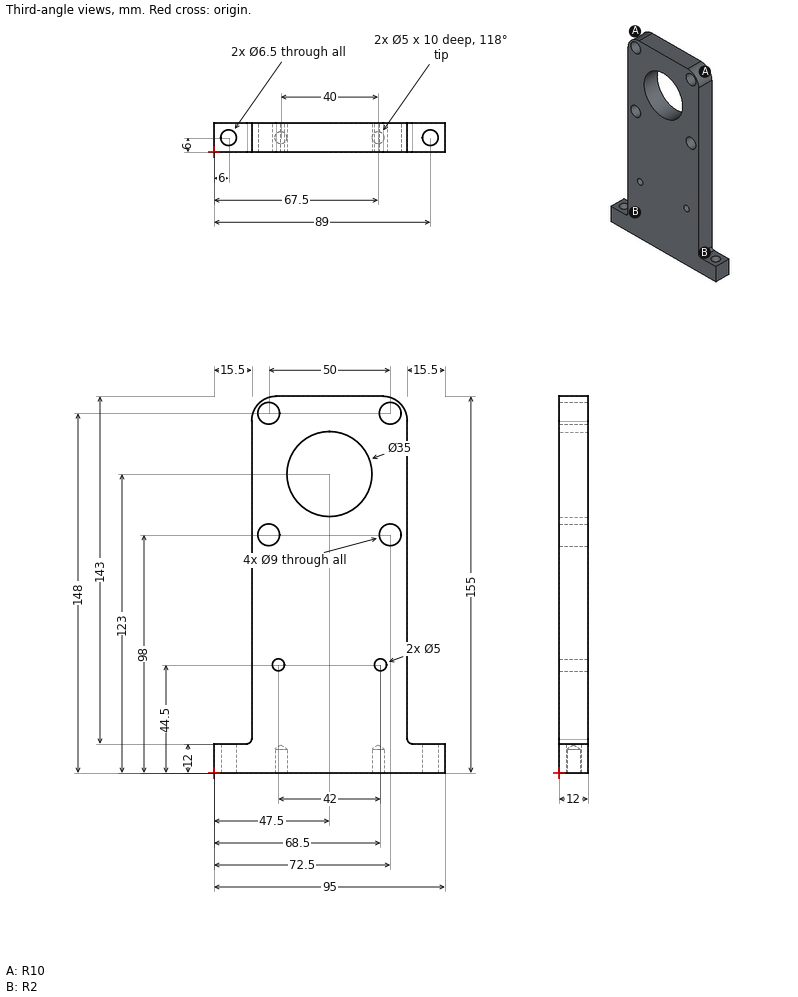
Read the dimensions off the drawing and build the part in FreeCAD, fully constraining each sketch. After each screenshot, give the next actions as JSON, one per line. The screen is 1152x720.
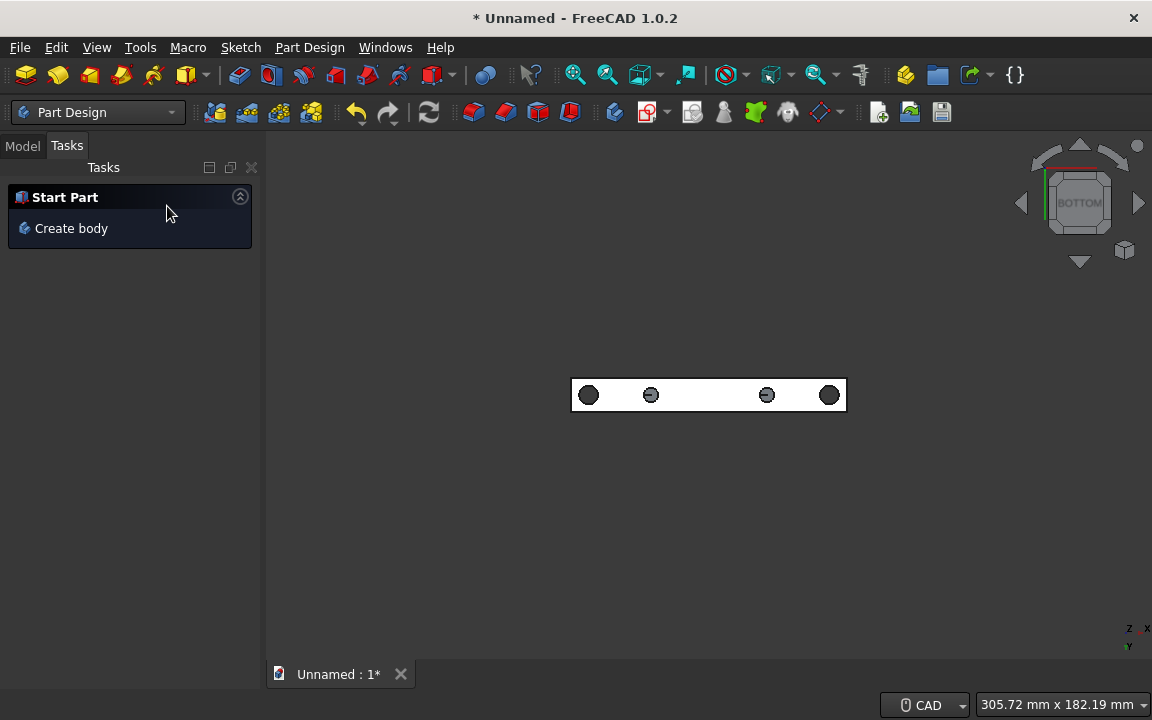
{"action": "key", "text": "0"}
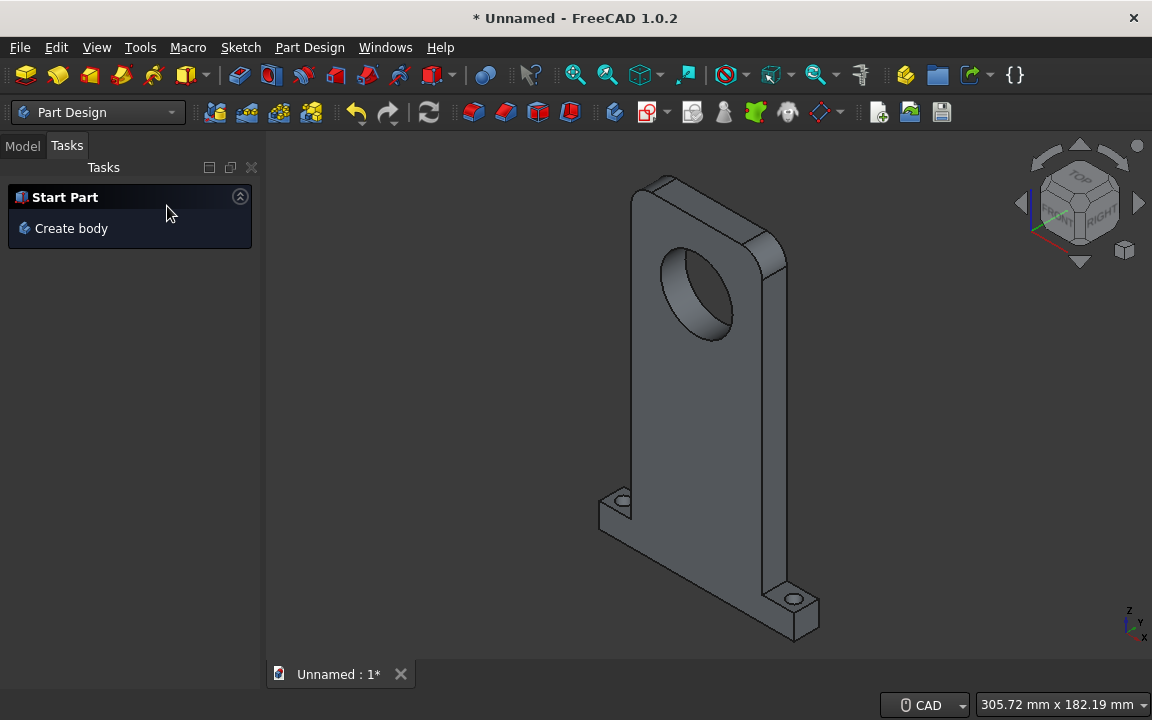
{"action": "key", "text": "2"}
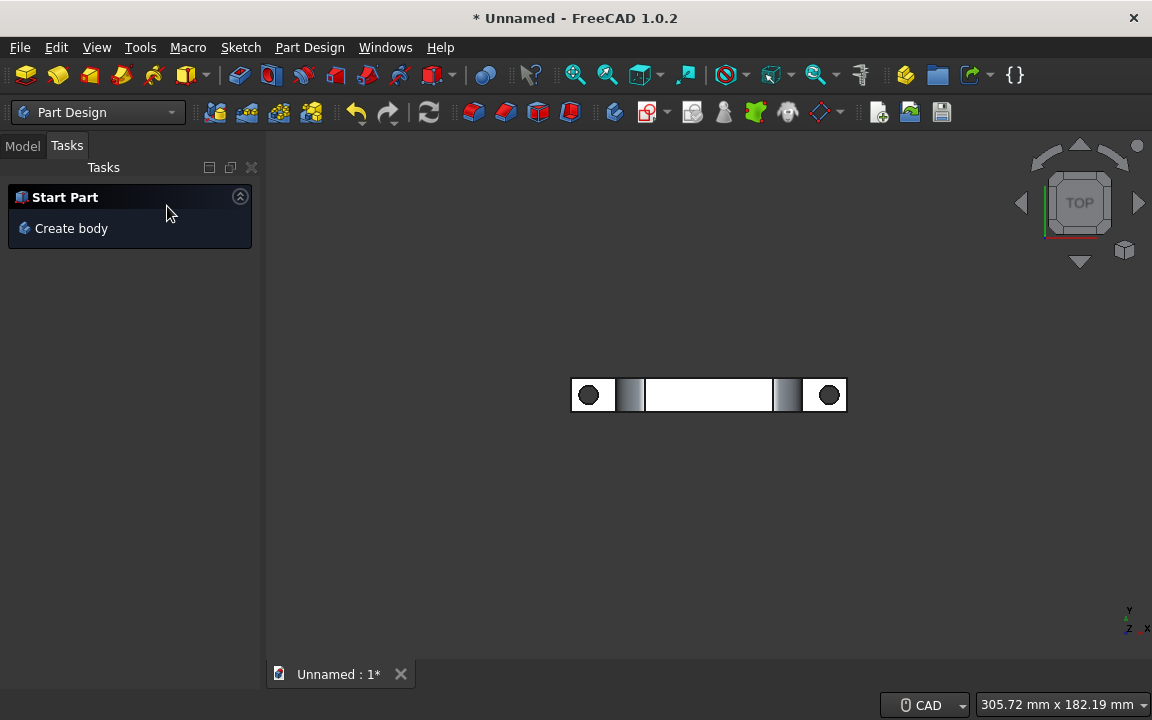
{"action": "left_click", "coordinate": [576, 76]}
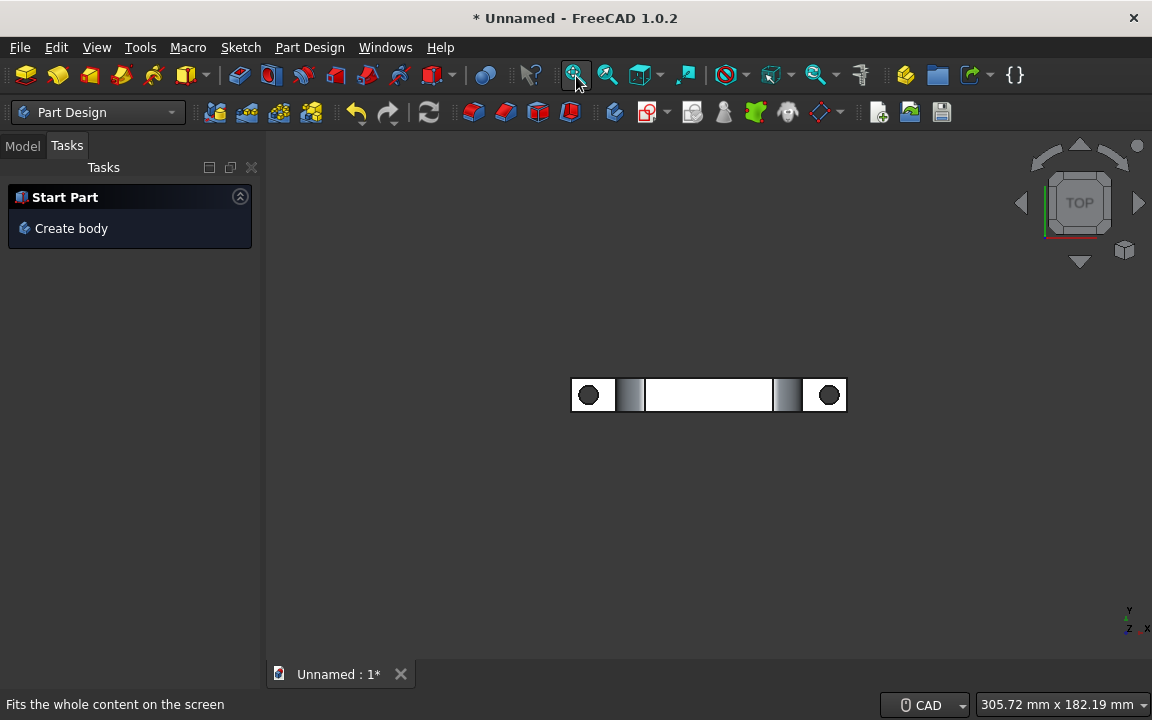
{"action": "key", "text": "1"}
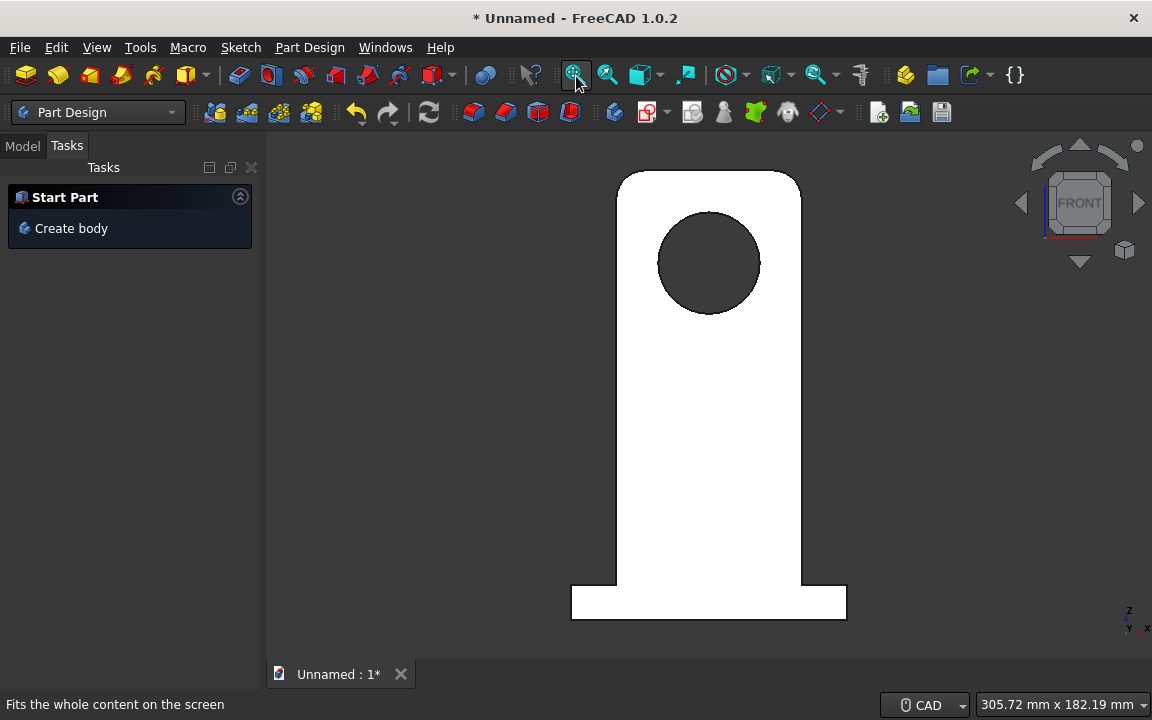
{"action": "key", "text": "3"}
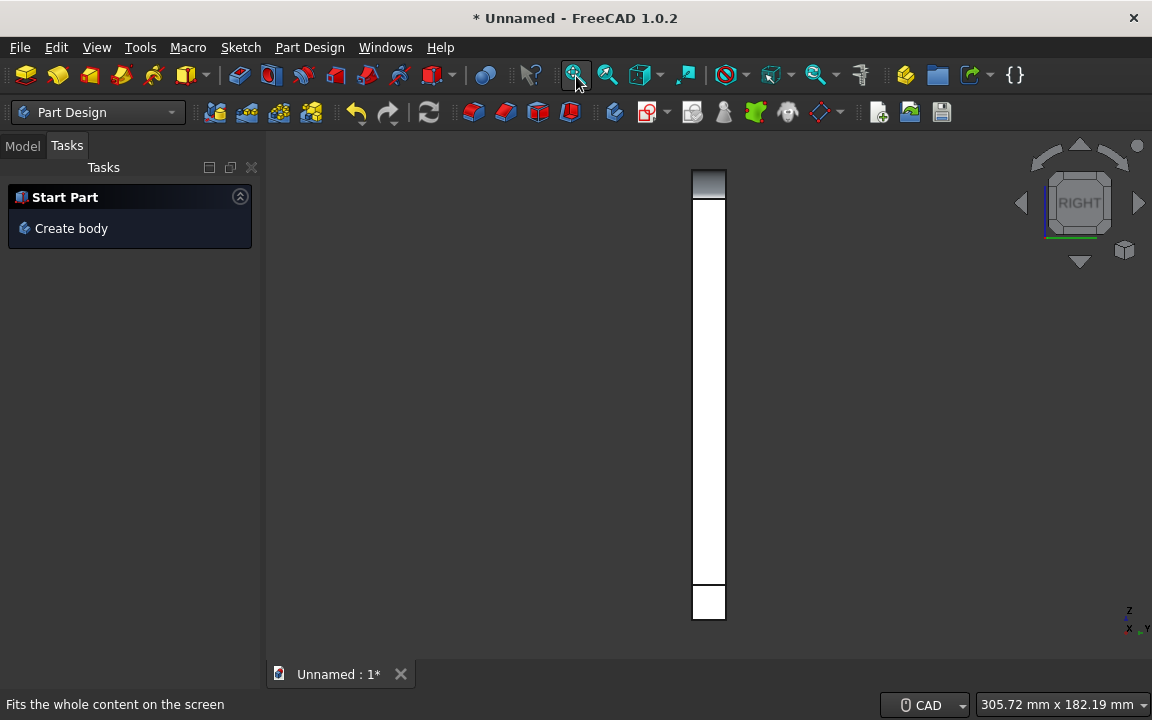
{"action": "key", "text": "5"}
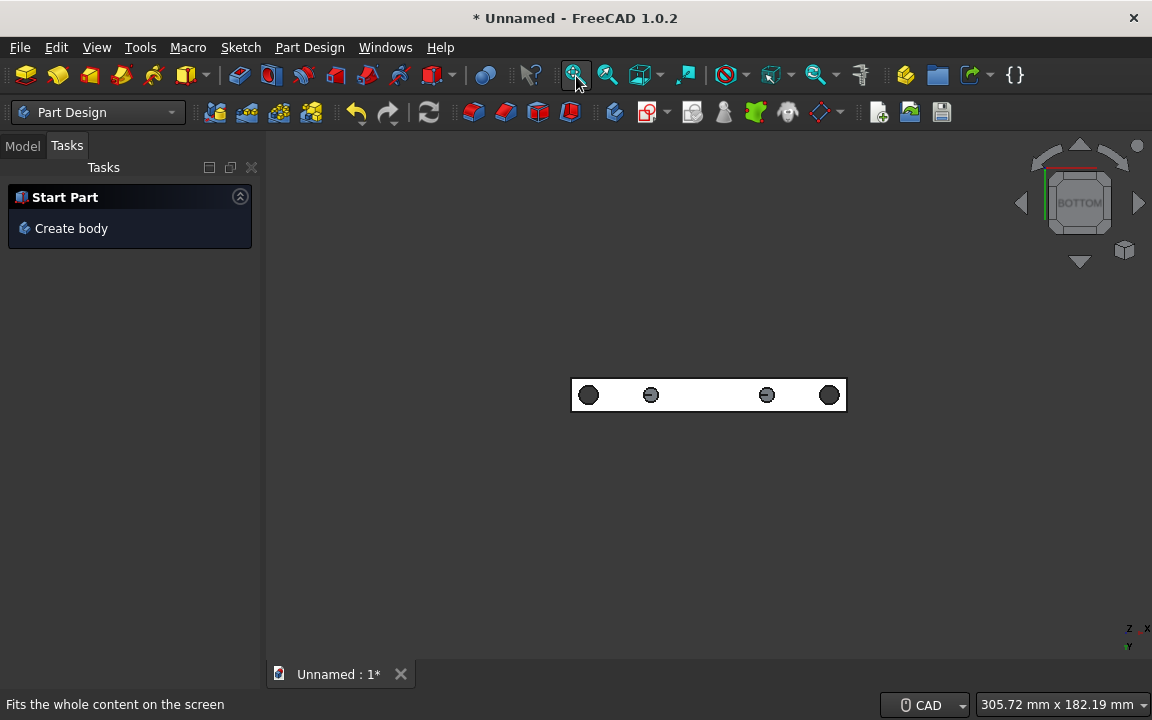
{"action": "key", "text": "v f"}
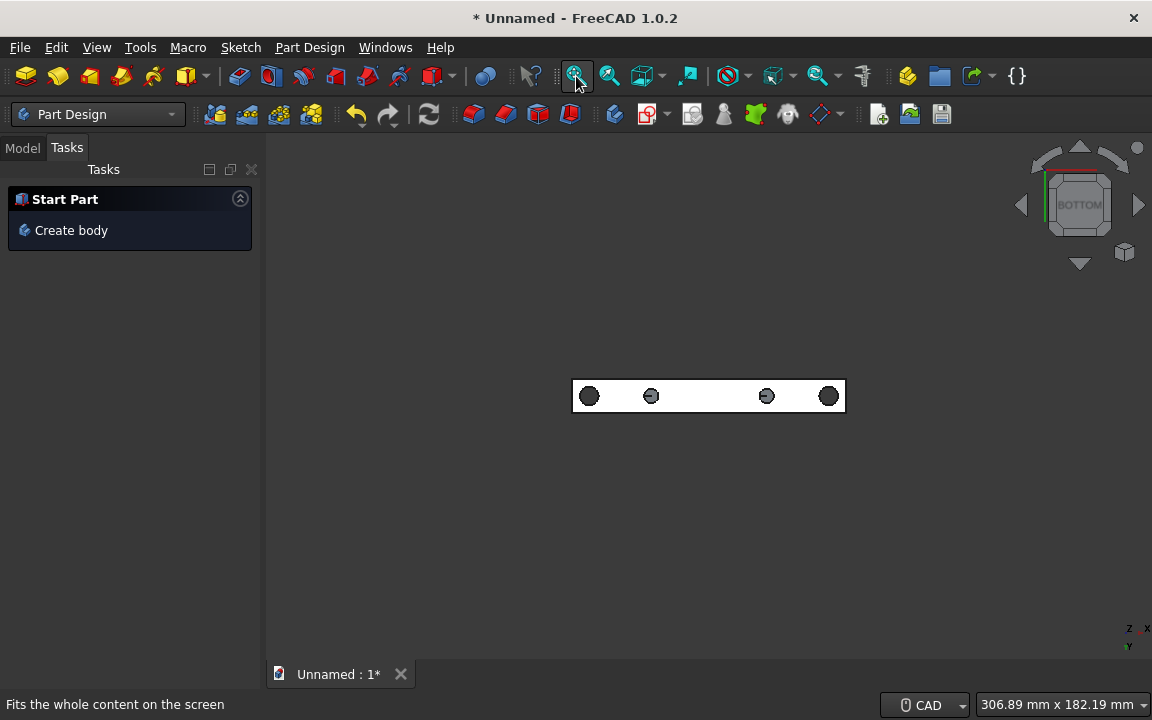
{"action": "key", "text": "4"}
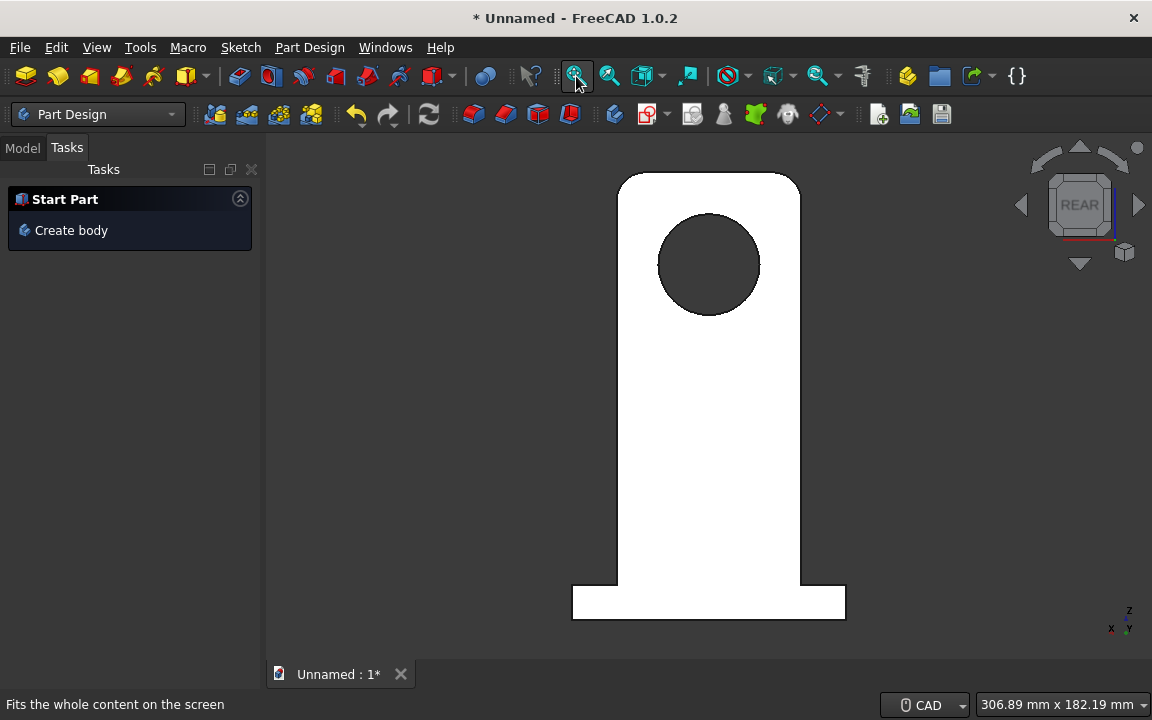
{"action": "key", "text": "6"}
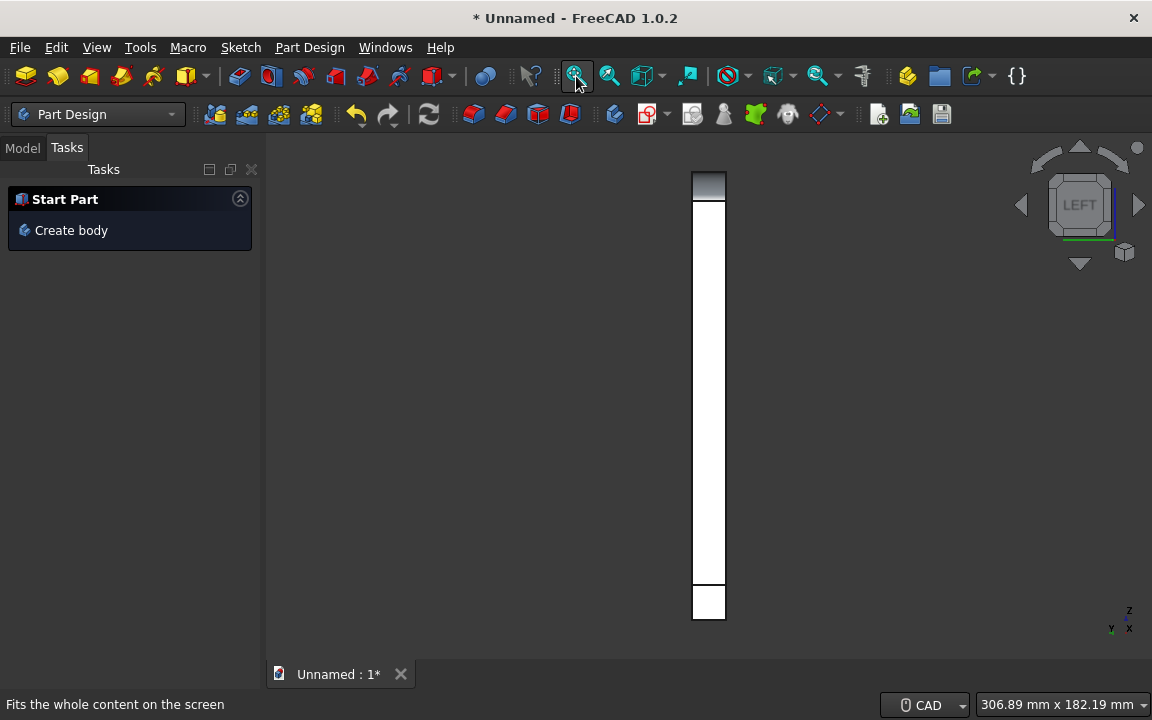
{"action": "key", "text": "v 3"}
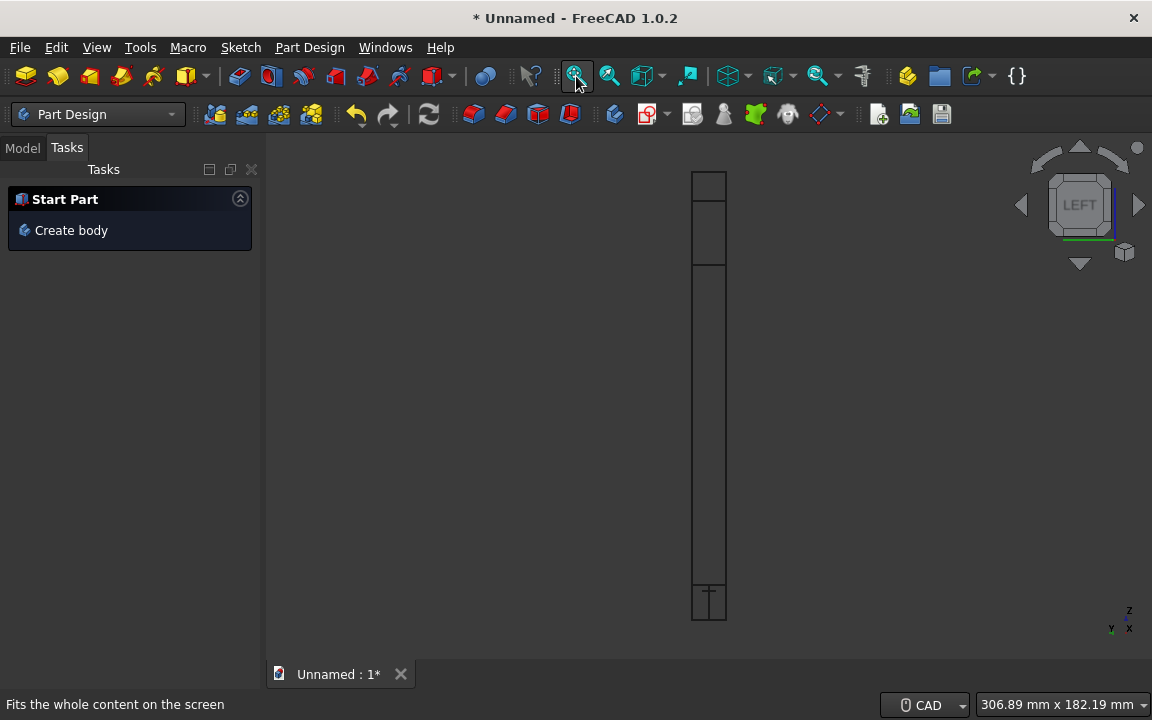
{"action": "key", "text": "0"}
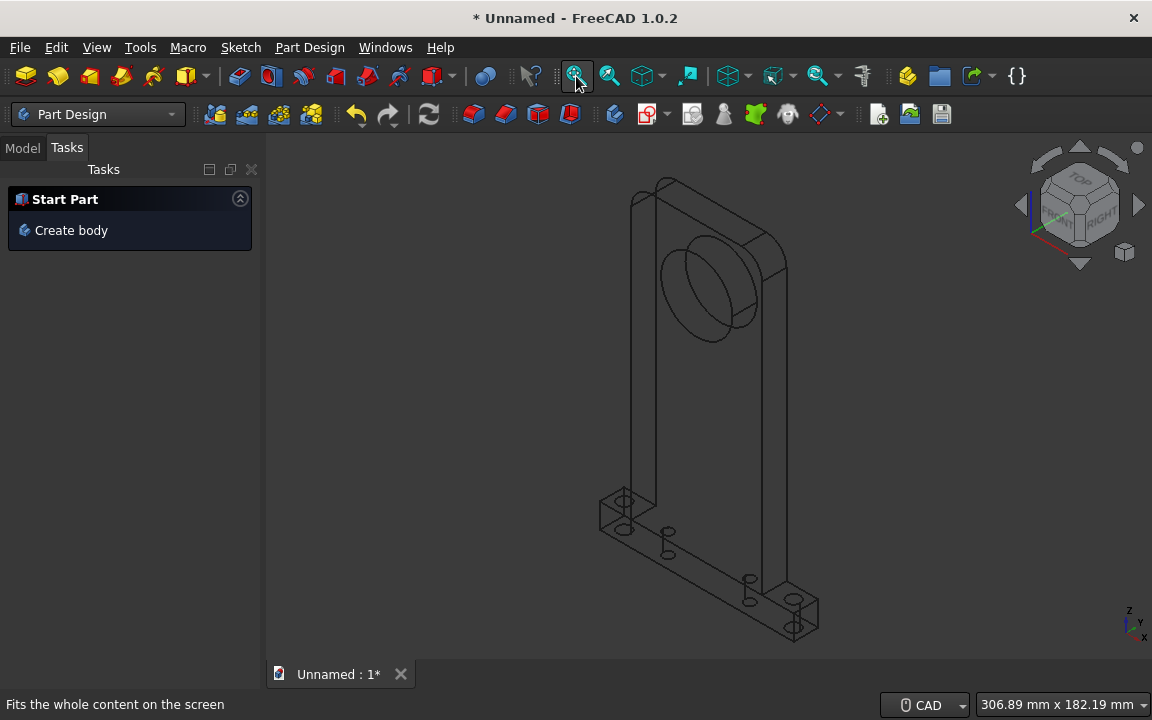
{"action": "left_click", "coordinate": [644, 512]}